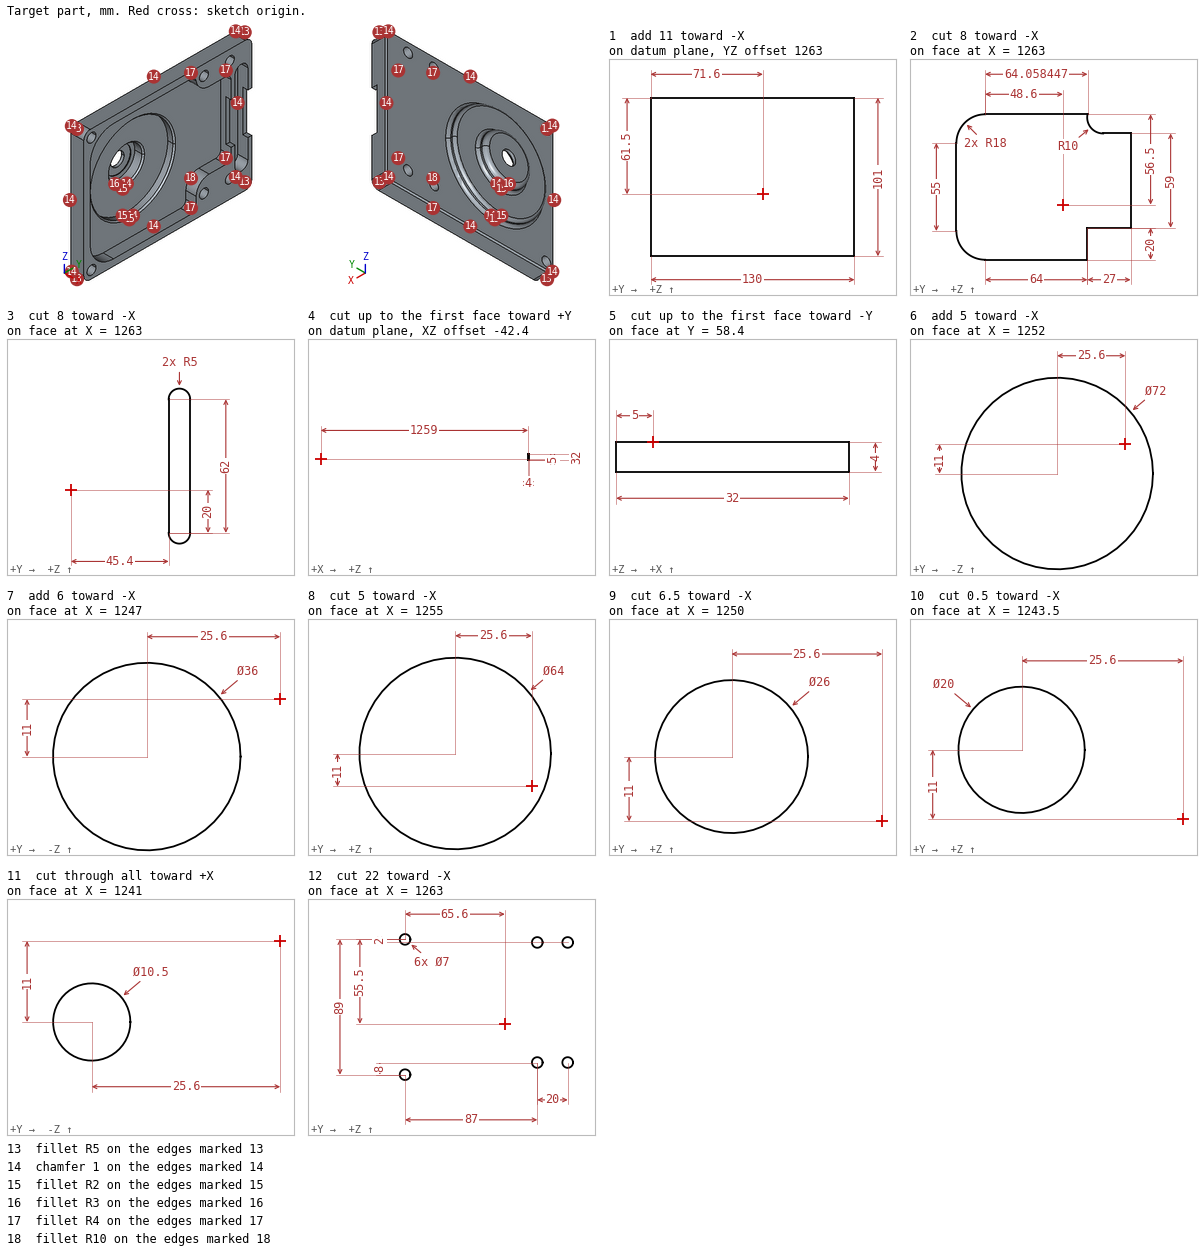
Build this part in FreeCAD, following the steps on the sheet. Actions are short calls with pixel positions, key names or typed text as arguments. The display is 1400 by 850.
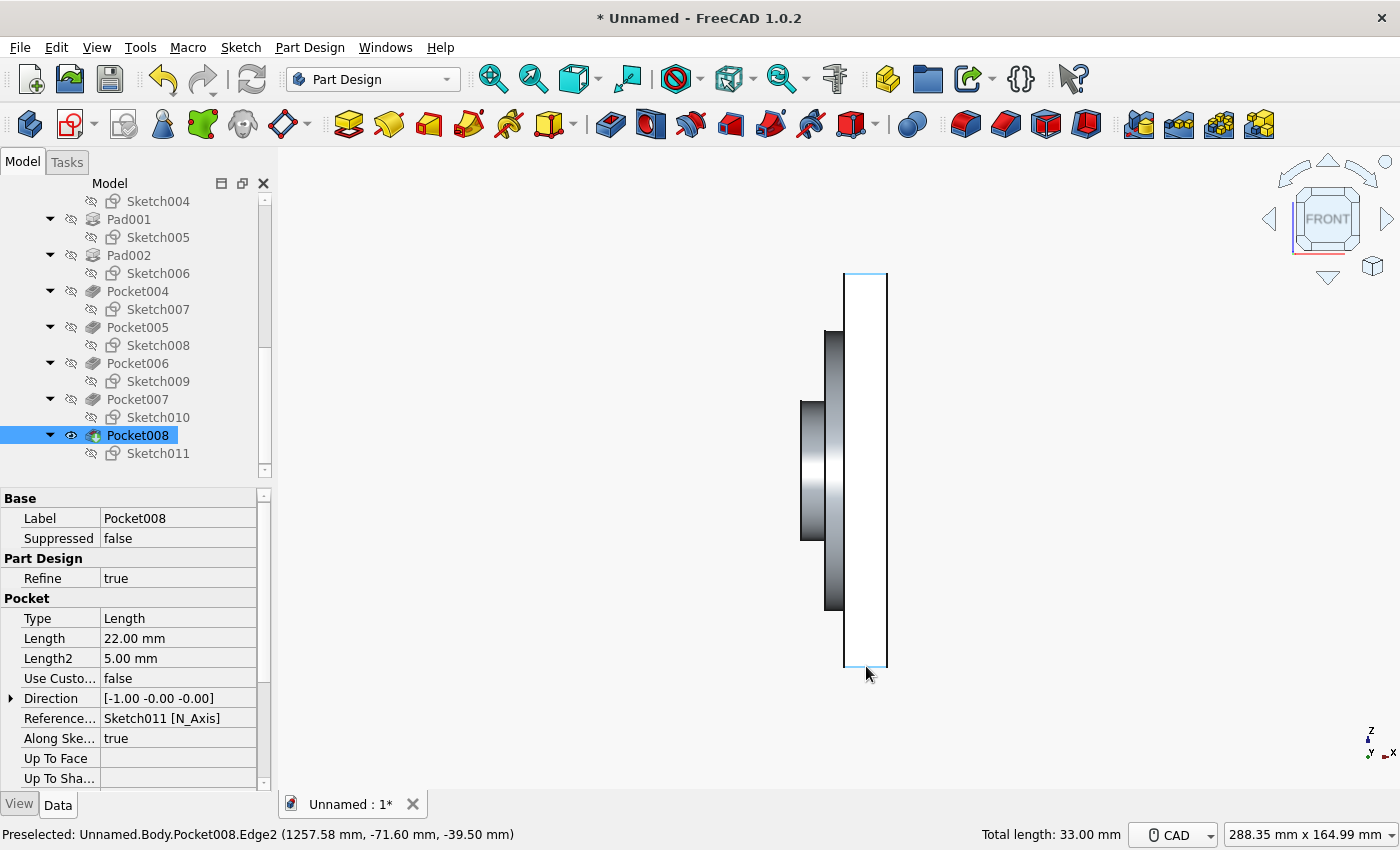
key(3)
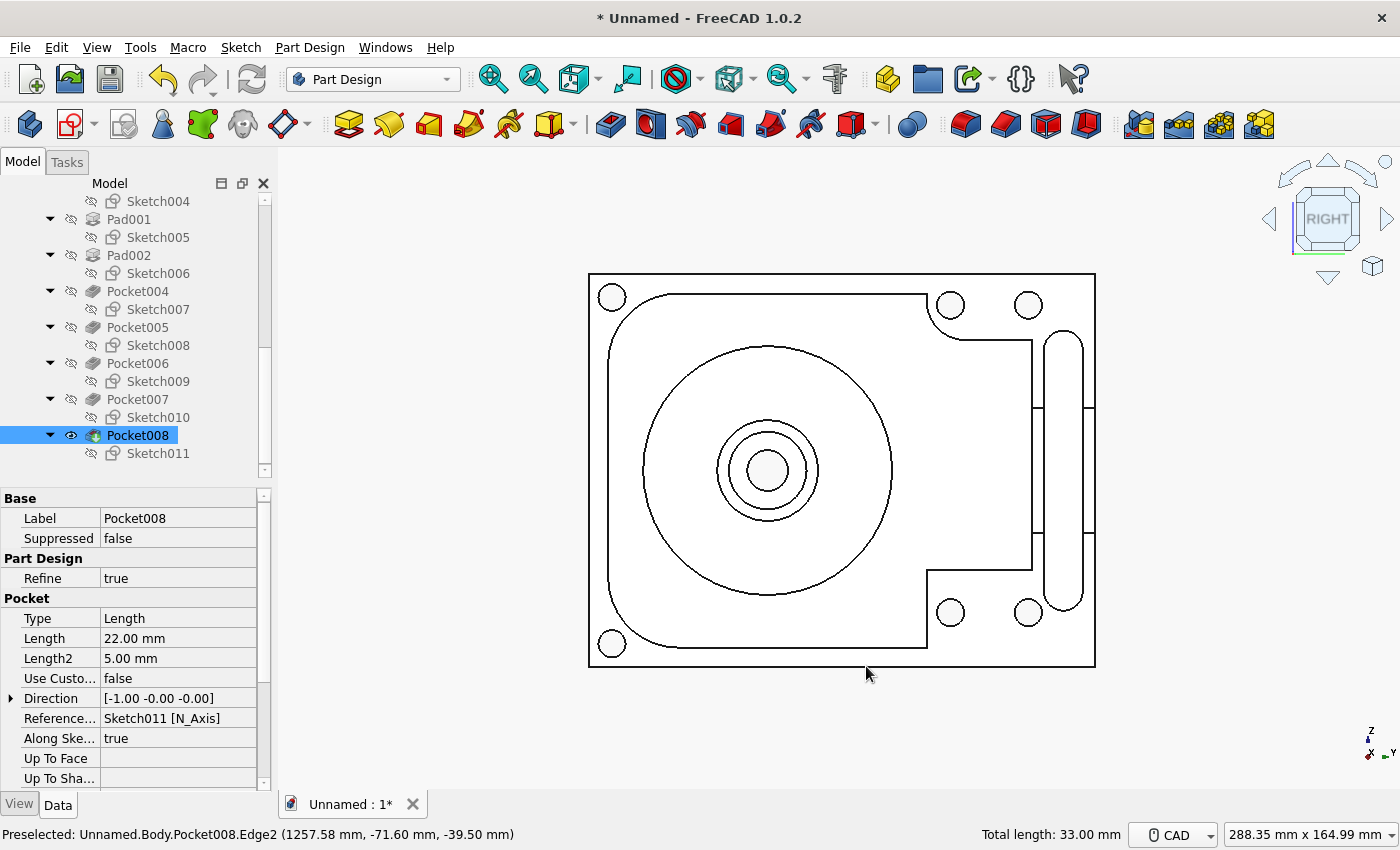
key(5)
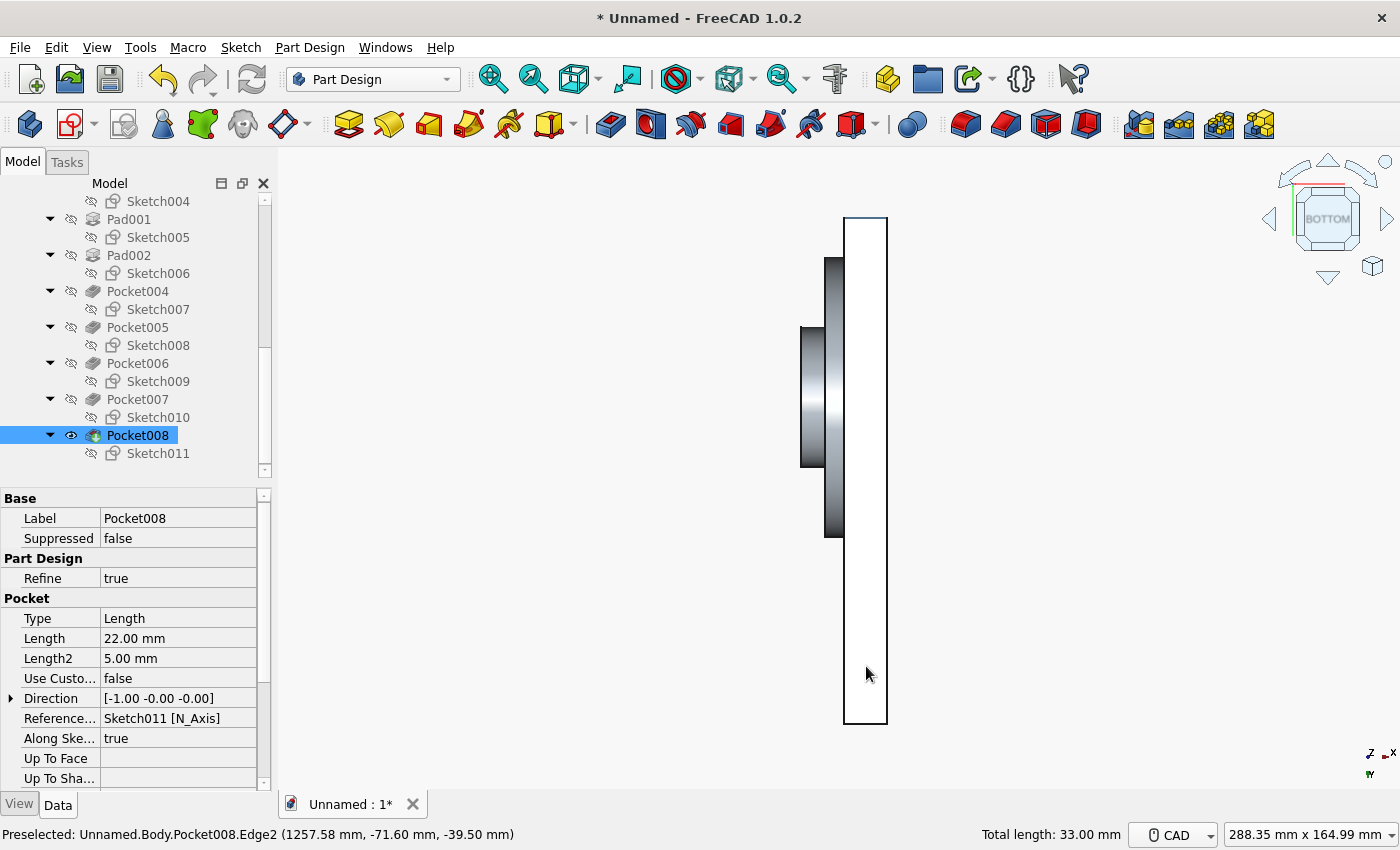
click(866, 723, ctrl)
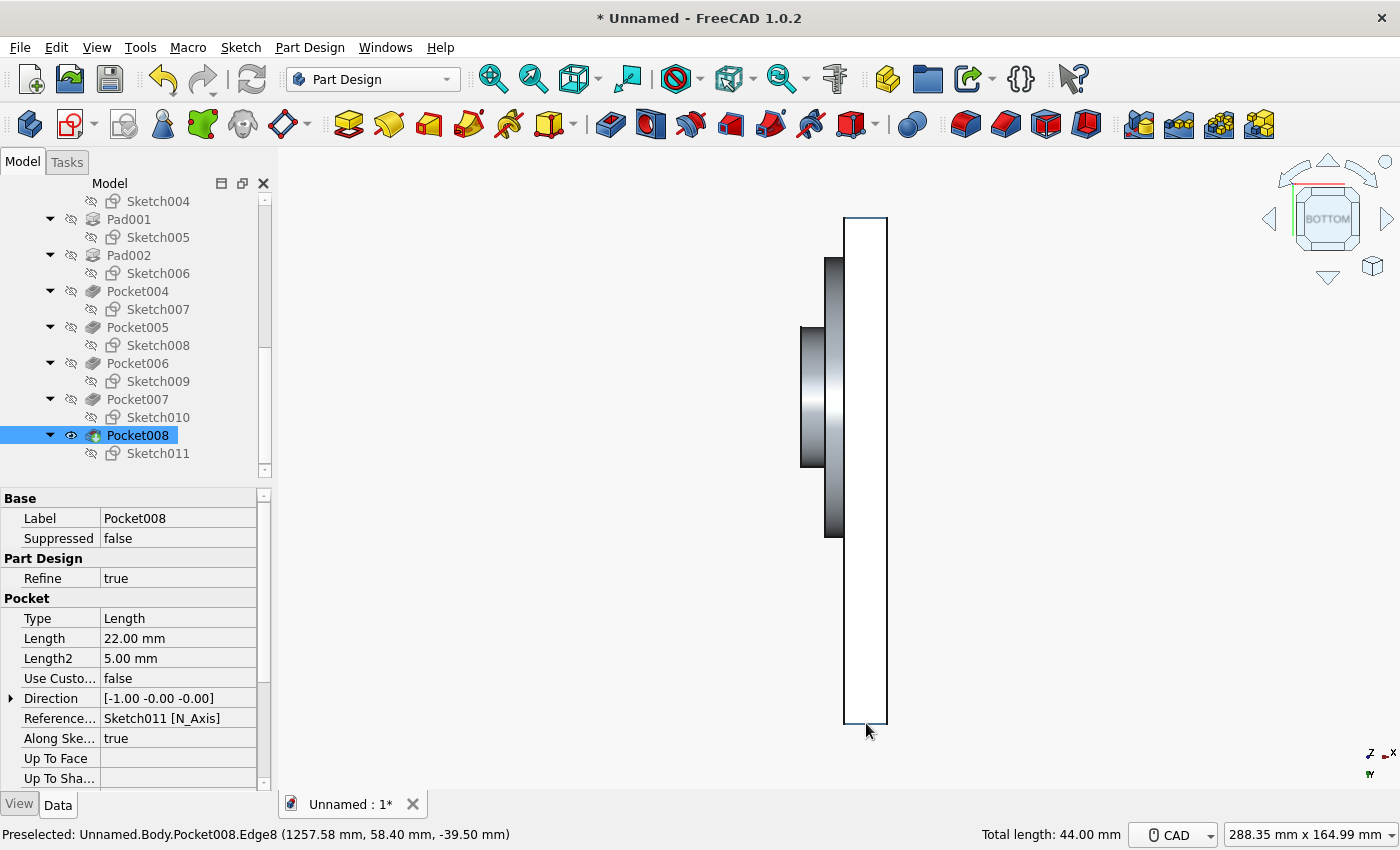
click(966, 124)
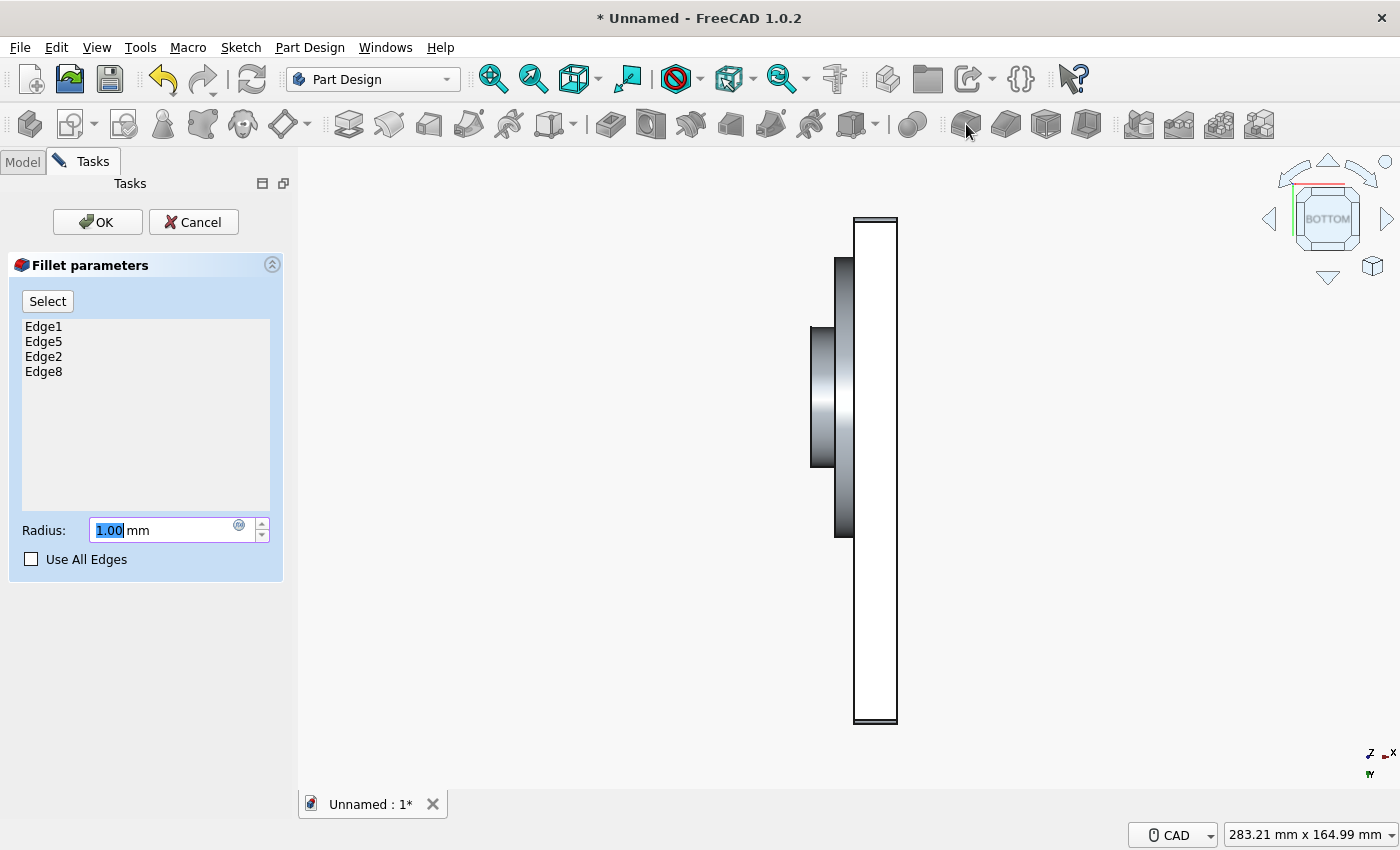
text(5)
key(Tab)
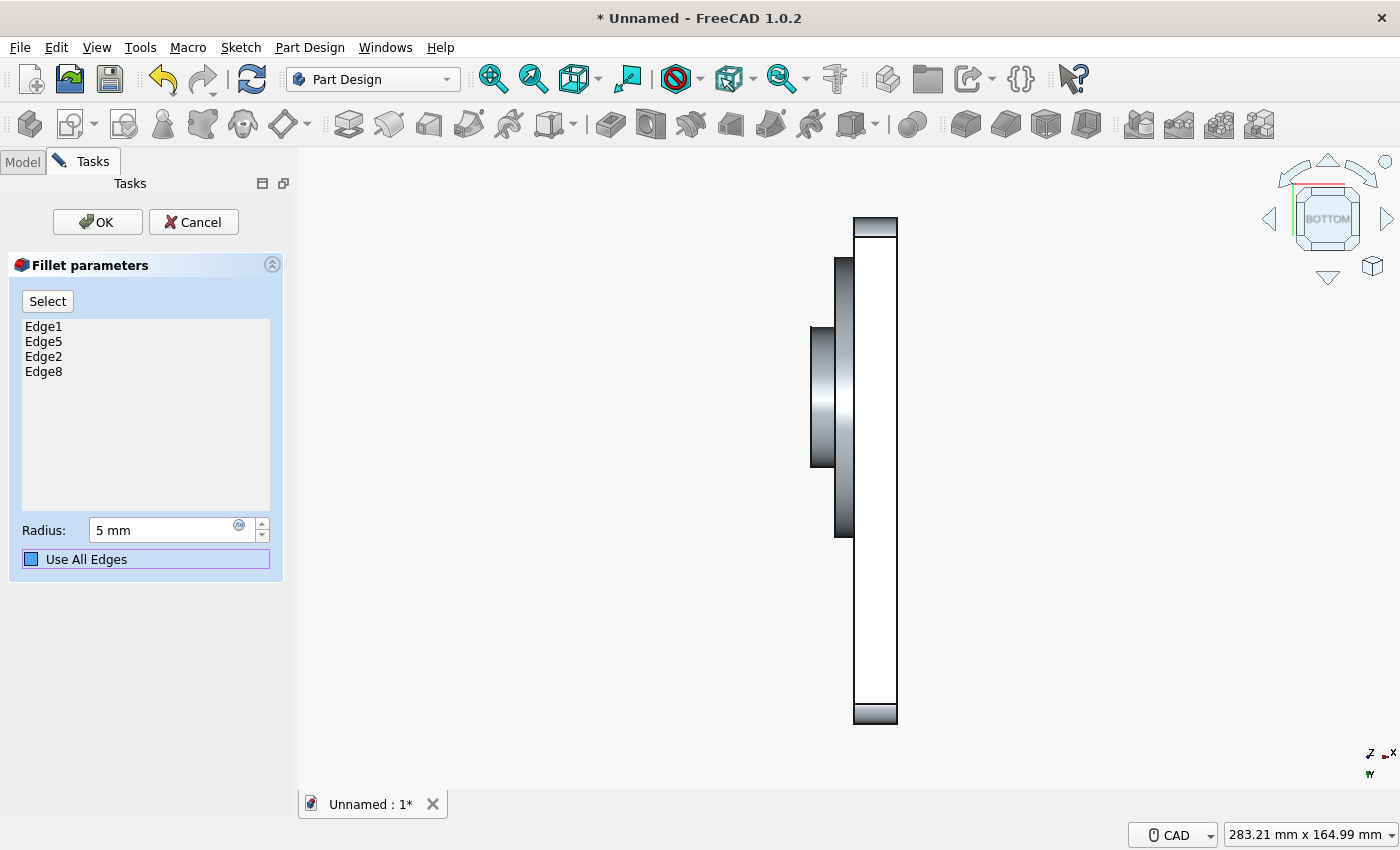
click(98, 222)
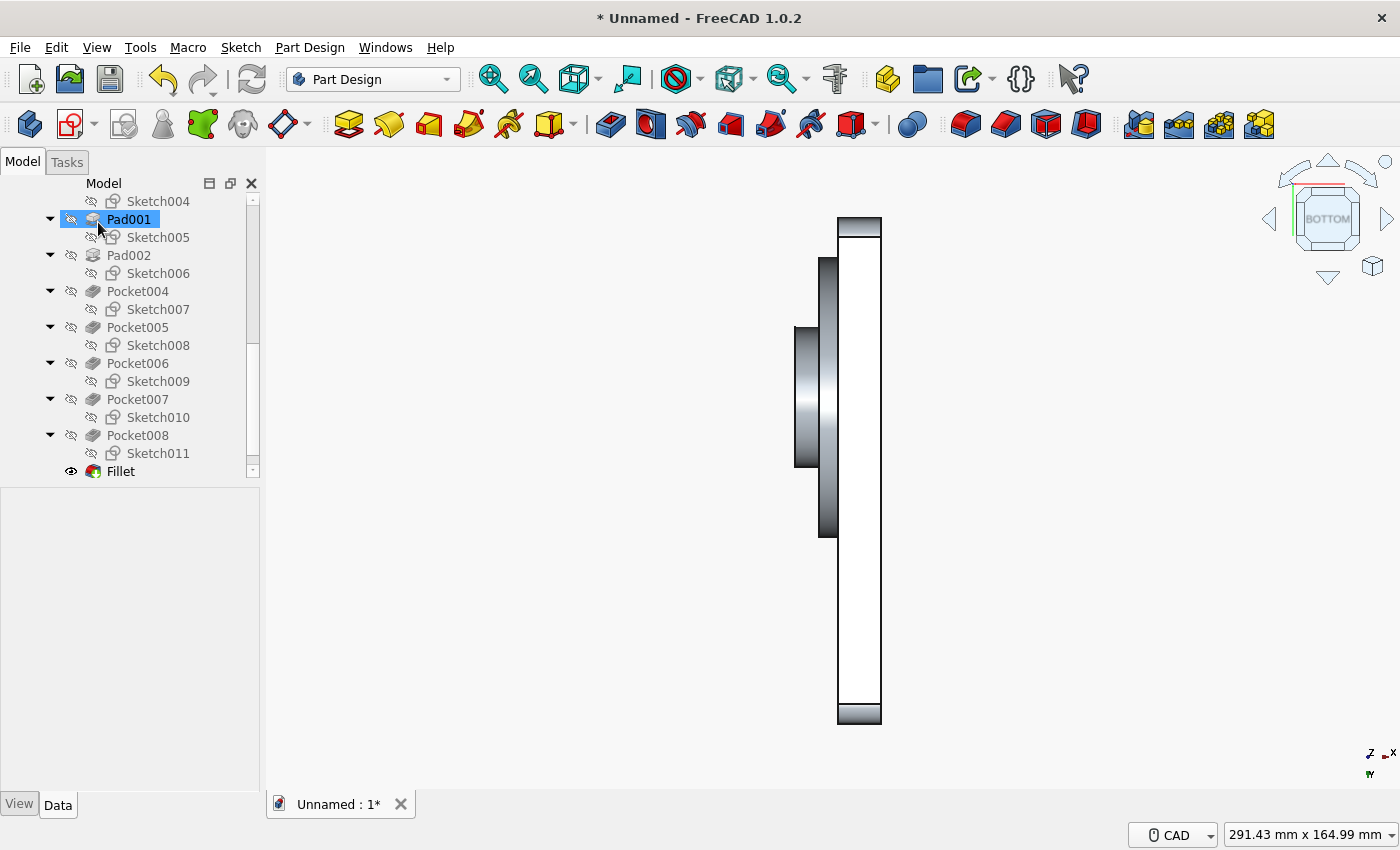
click(838, 470)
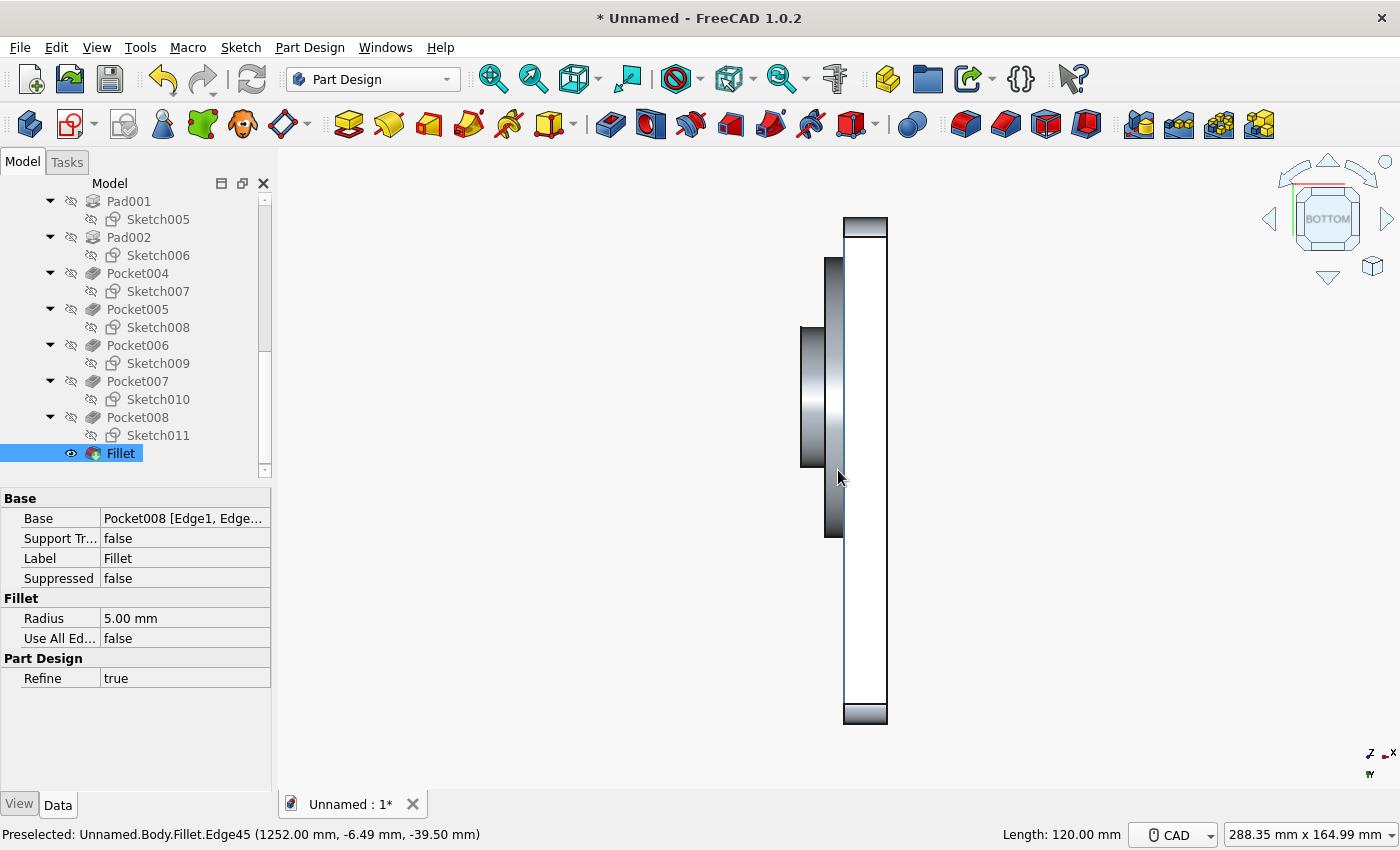
click(844, 222, ctrl)